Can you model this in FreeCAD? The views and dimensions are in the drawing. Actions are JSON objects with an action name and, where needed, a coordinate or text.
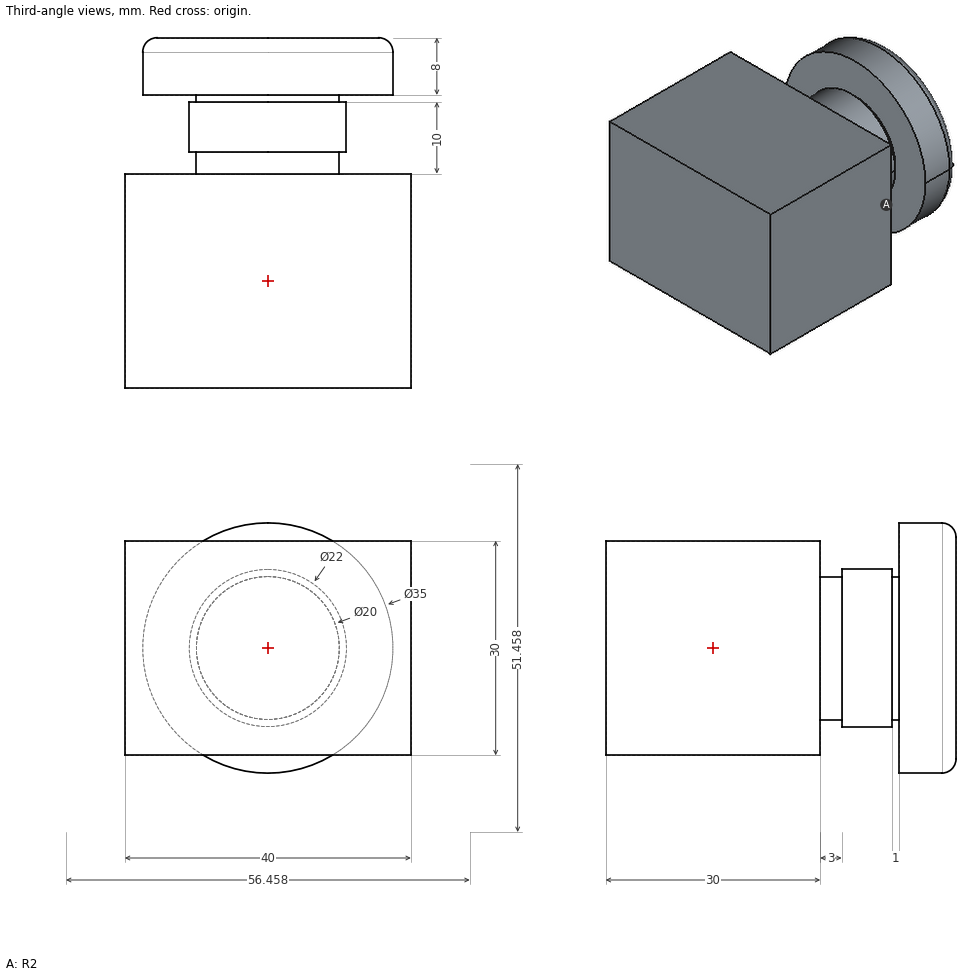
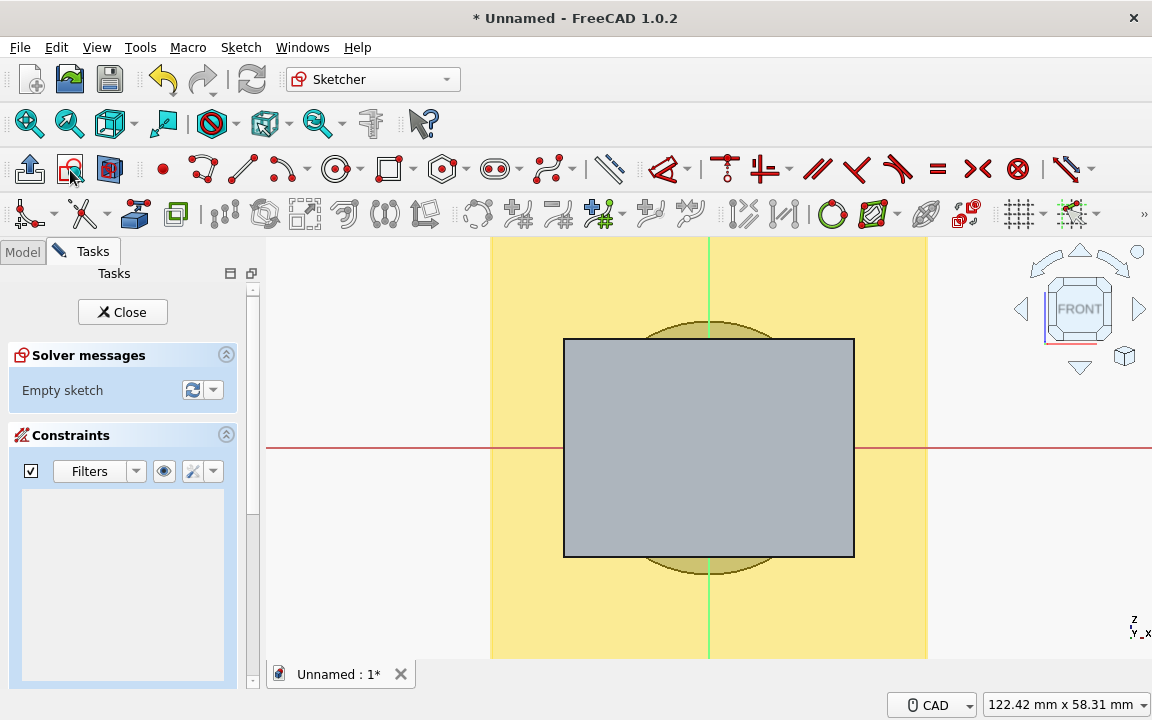
{"action": "left_click", "coordinate": [110, 170]}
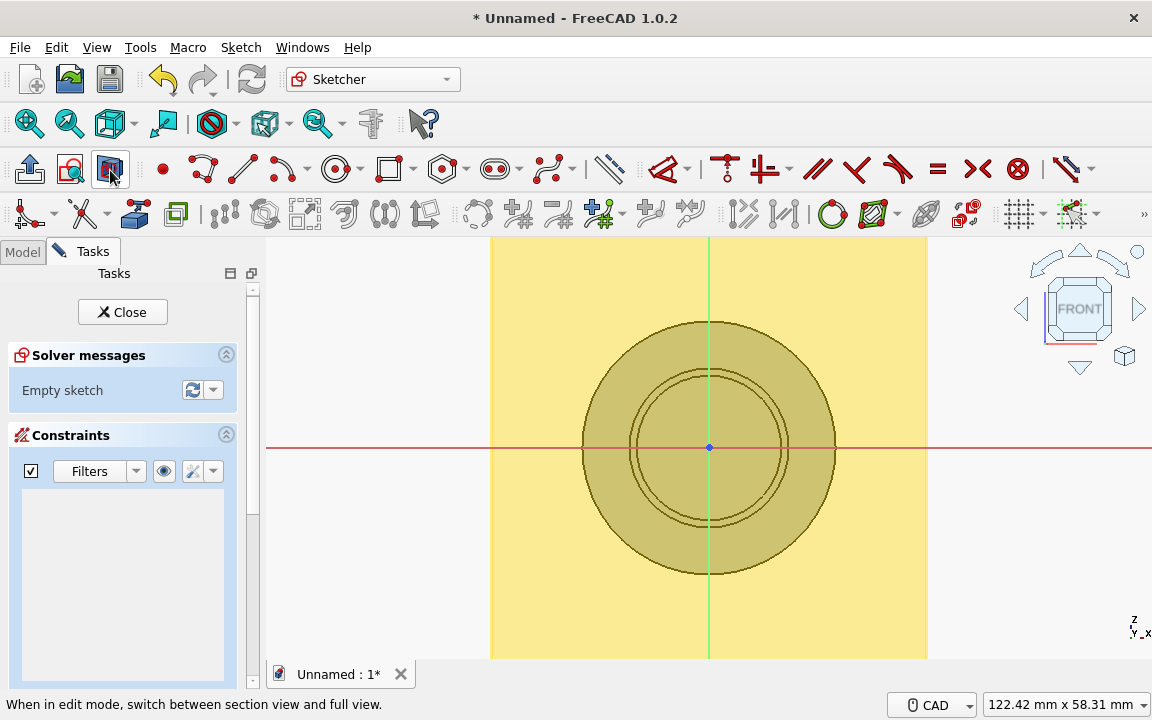
{"action": "scroll", "coordinate": [501, 448], "scroll_direction": "down", "scroll_amount": 2}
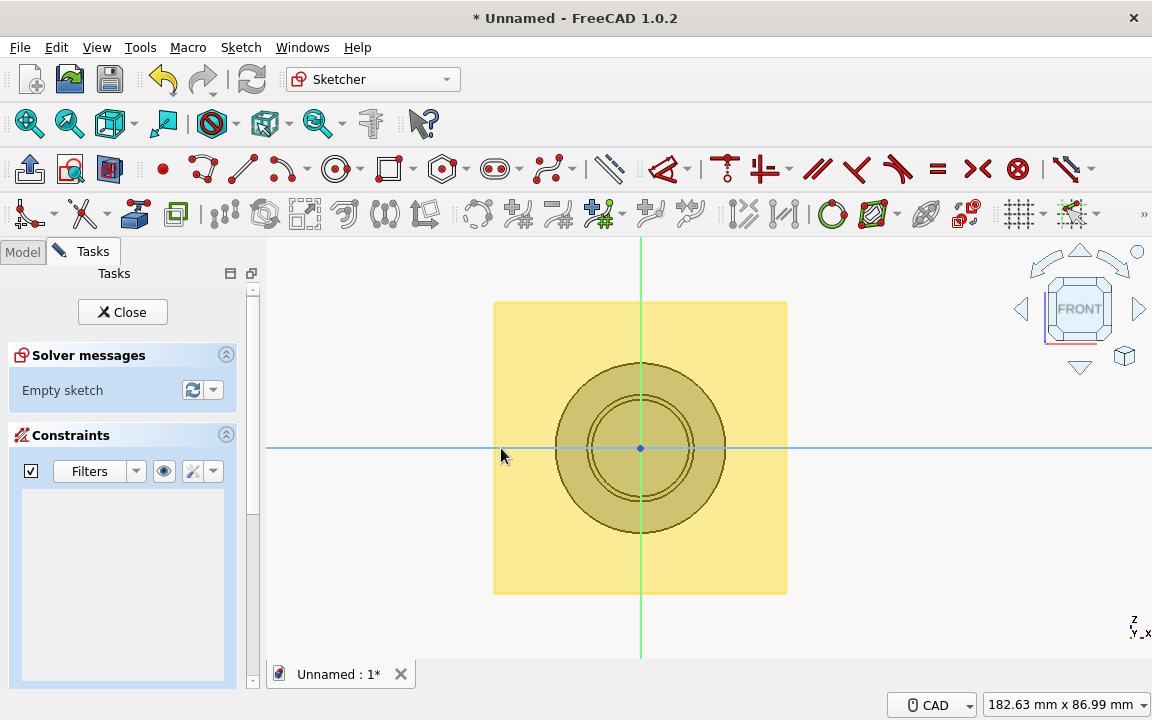
{"action": "left_click", "coordinate": [416, 170]}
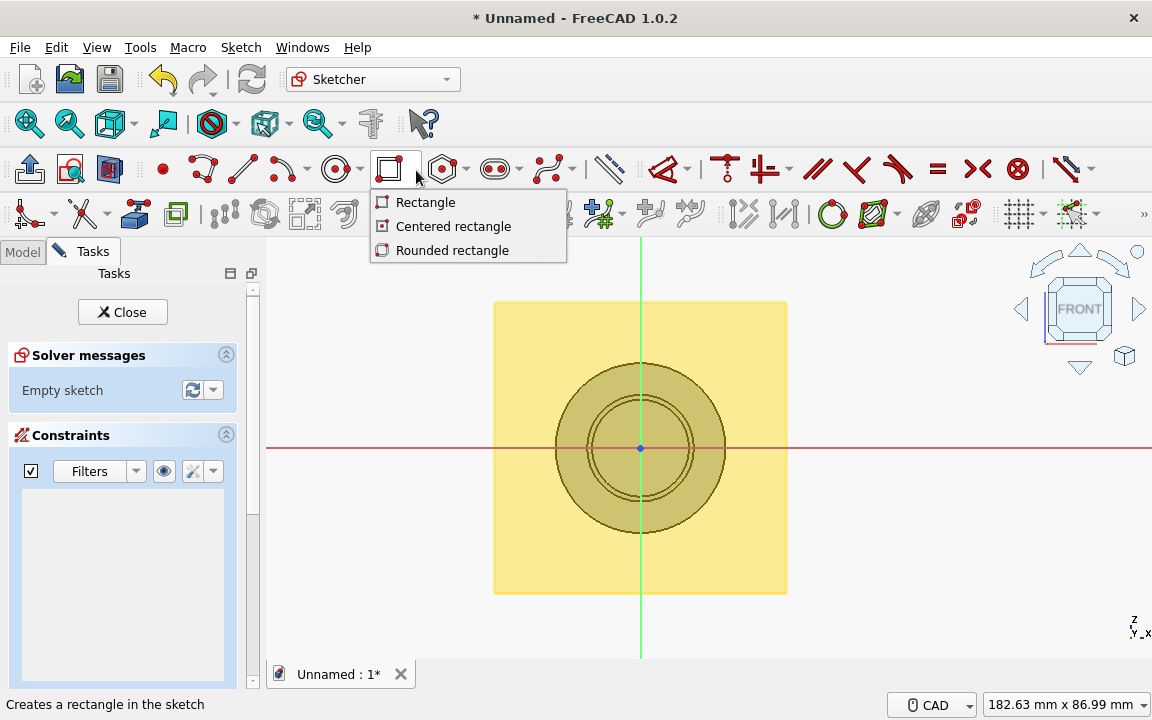
{"action": "left_click", "coordinate": [468, 226]}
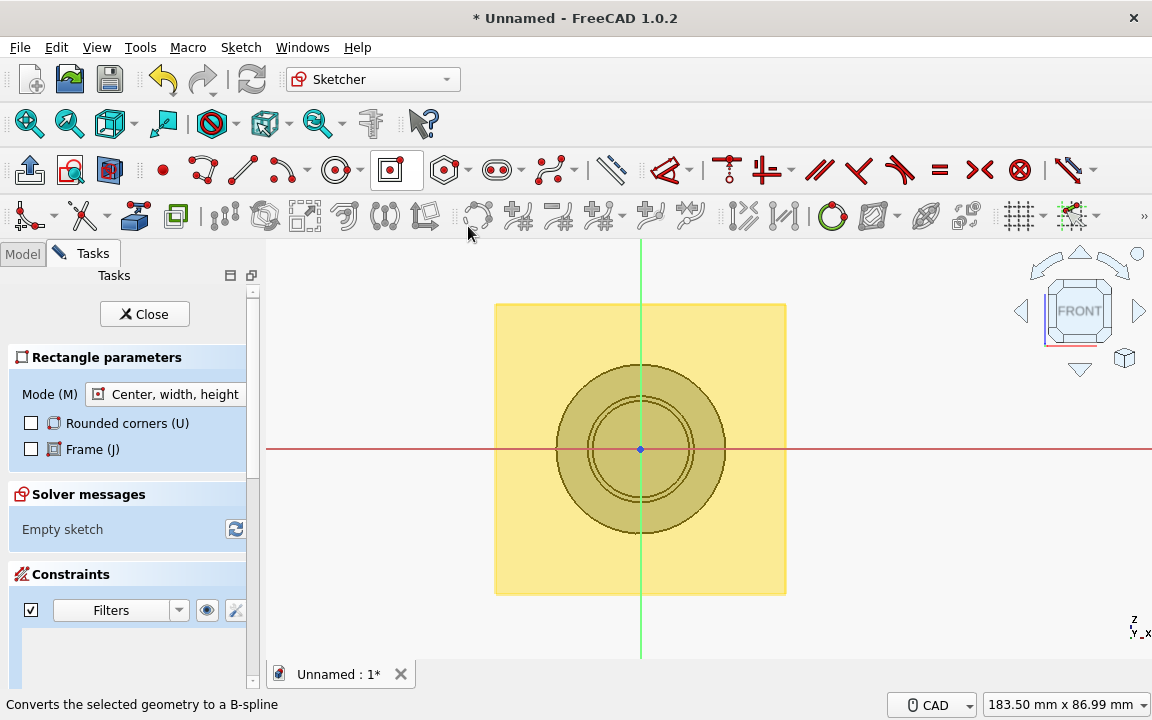
{"action": "left_click", "coordinate": [641, 449]}
{"action": "mouse_move", "coordinate": [777, 325]}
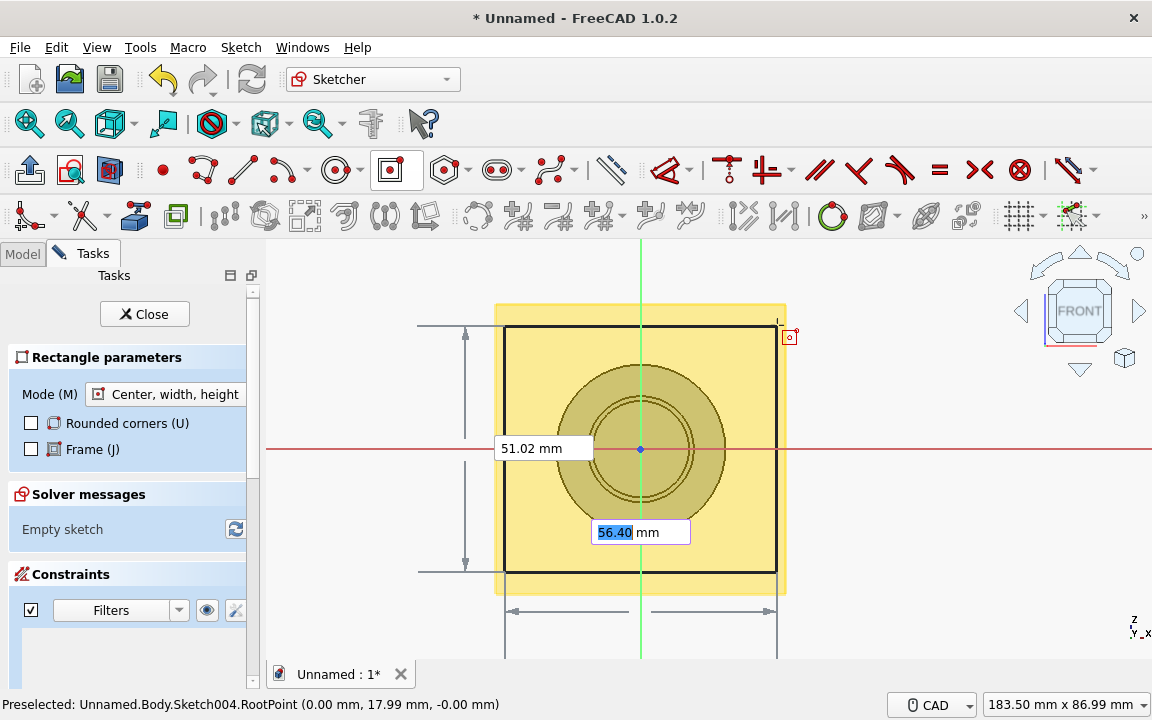
{"action": "type", "text": "56.458"}
{"action": "key", "text": "Tab"}
{"action": "type", "text": "51.458"}
{"action": "key", "text": "Return"}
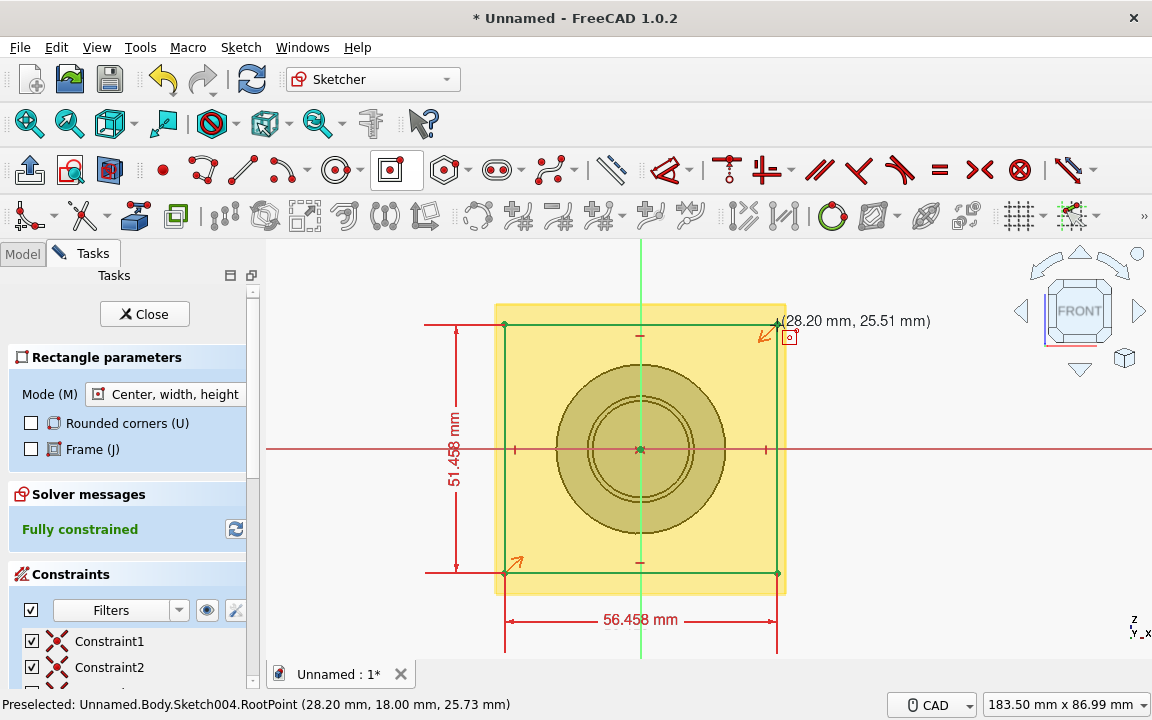
{"action": "left_click", "coordinate": [336, 170]}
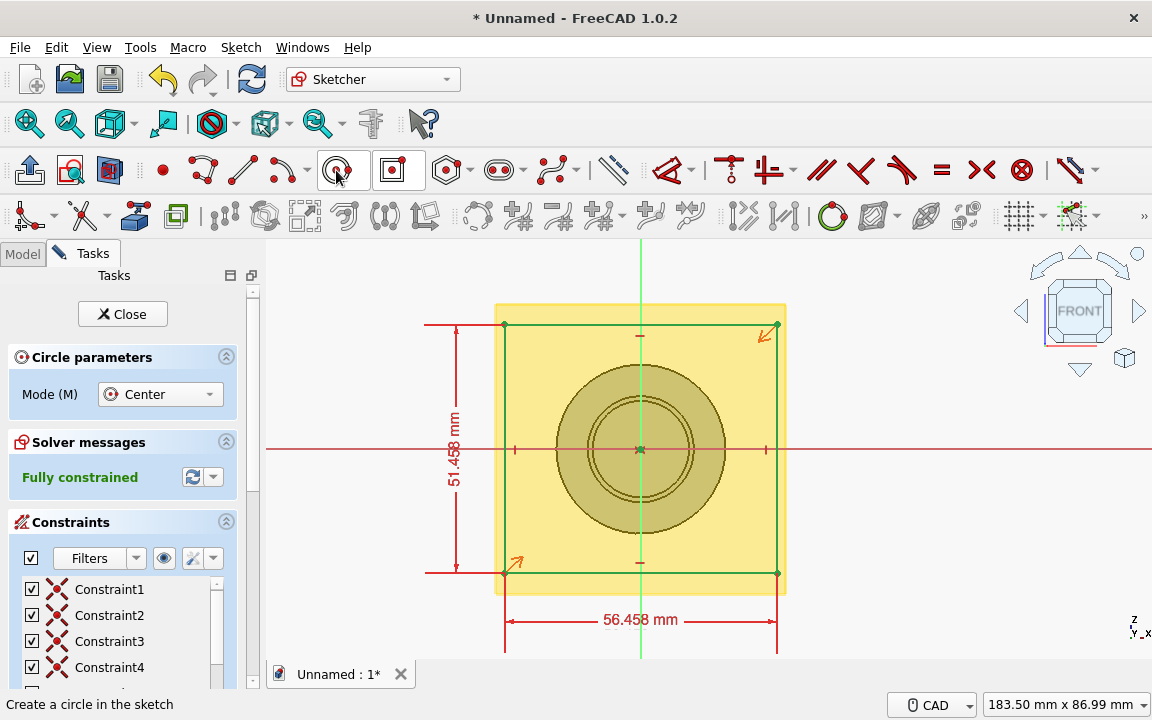
{"action": "left_click", "coordinate": [641, 449]}
{"action": "mouse_move", "coordinate": [675, 415]}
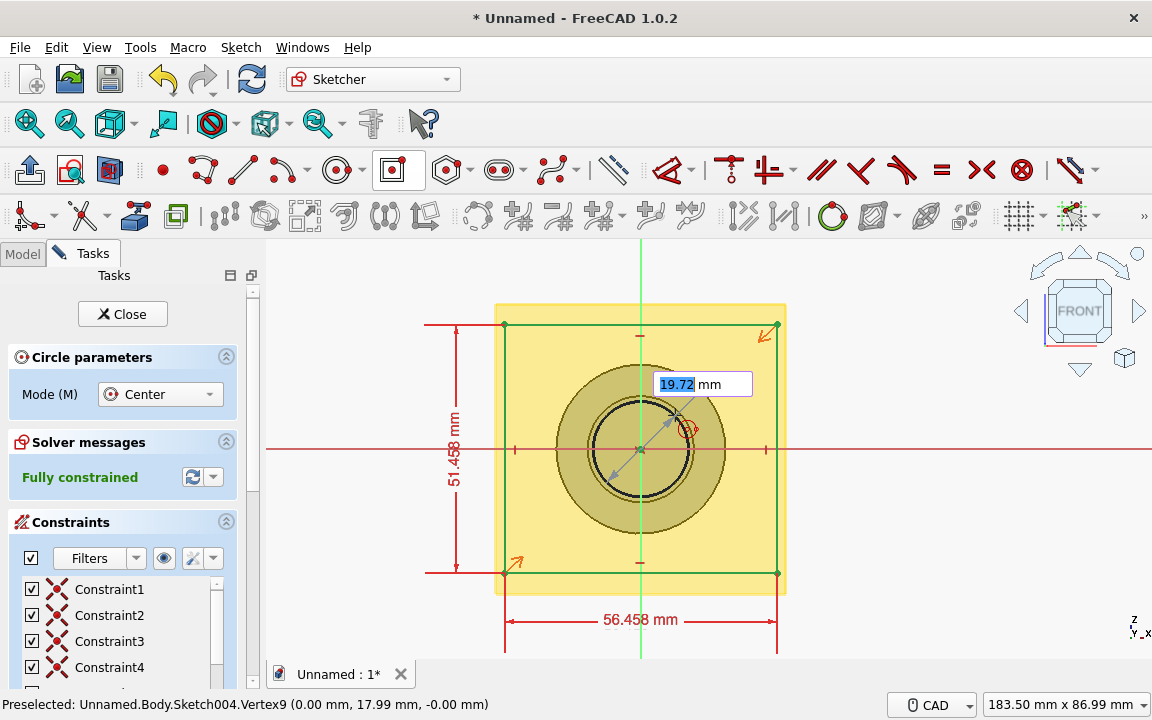
{"action": "type", "text": "20"}
{"action": "key", "text": "Return"}
{"action": "key", "text": "Escape"}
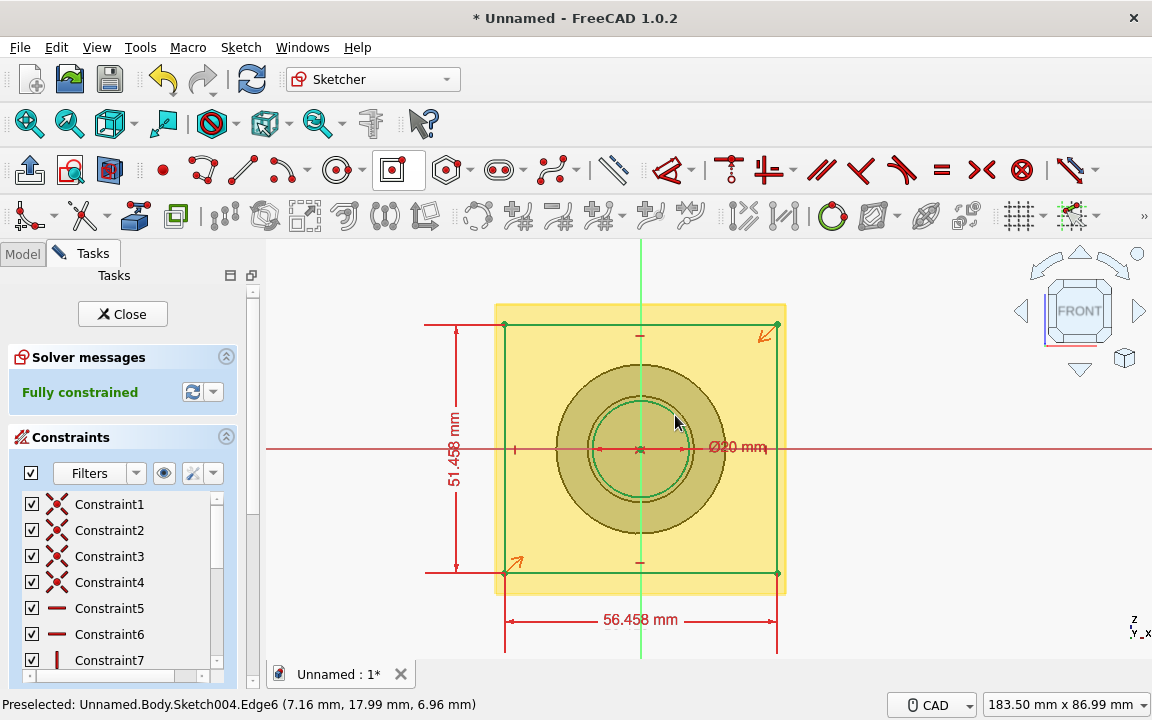
{"action": "left_click", "coordinate": [123, 314]}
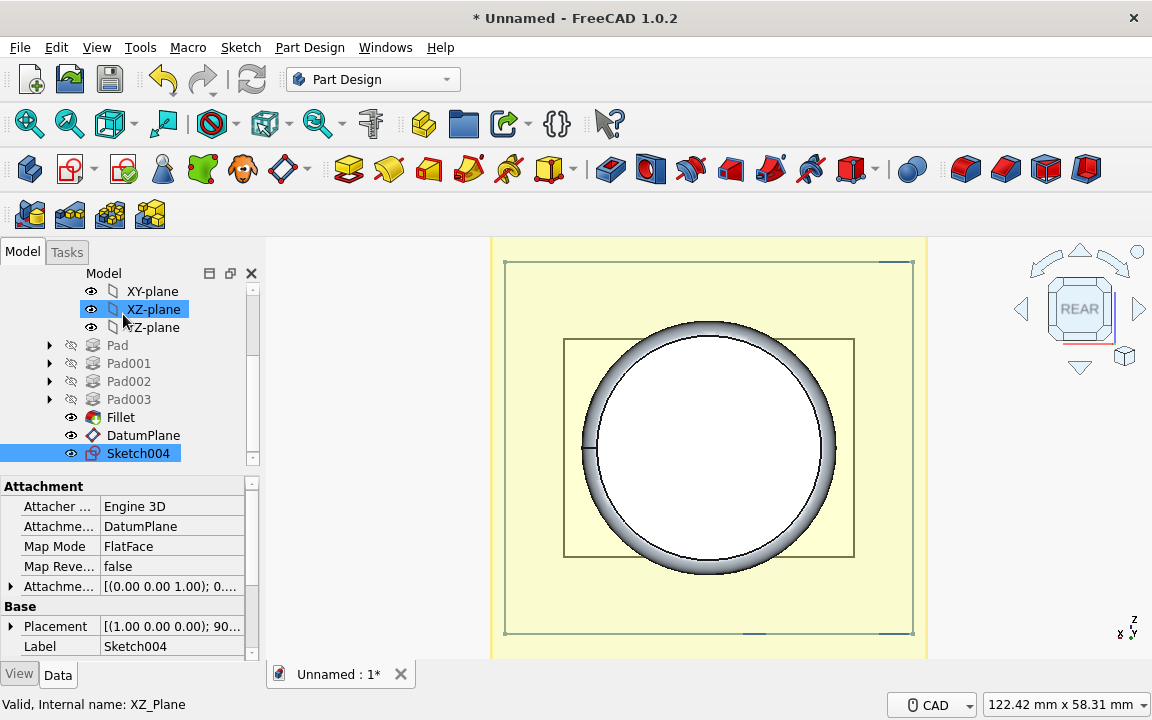
{"action": "left_click", "coordinate": [612, 170]}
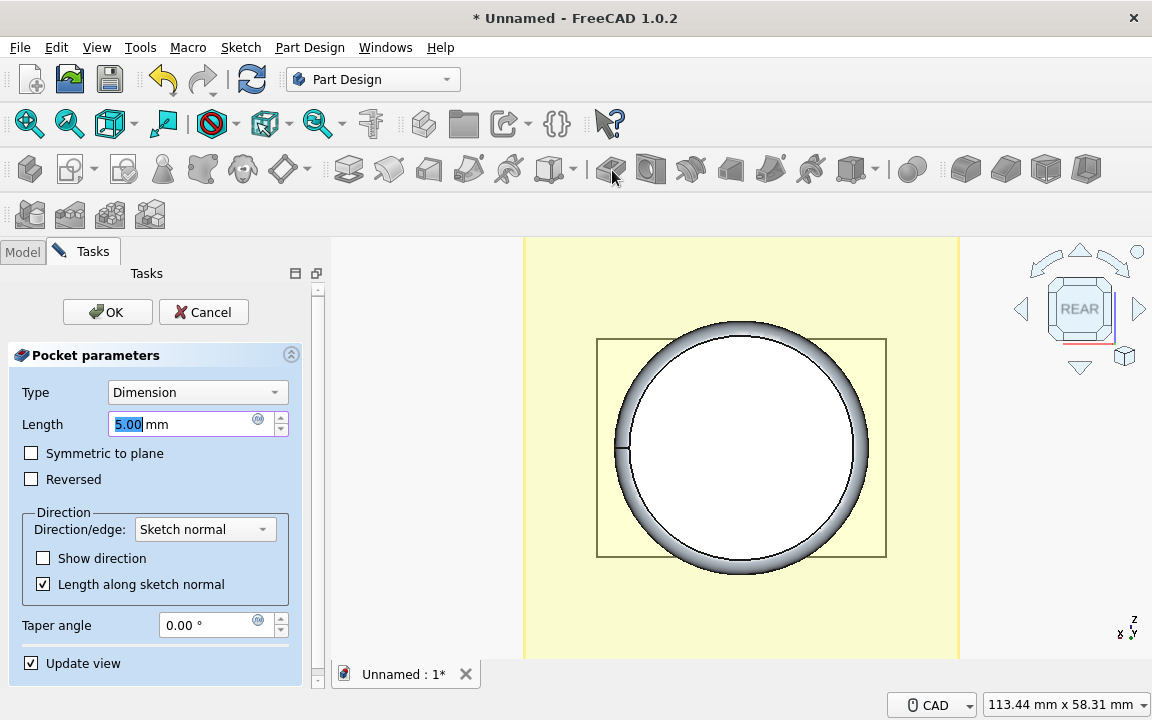
{"action": "type", "text": "3"}
{"action": "key", "text": "Tab"}